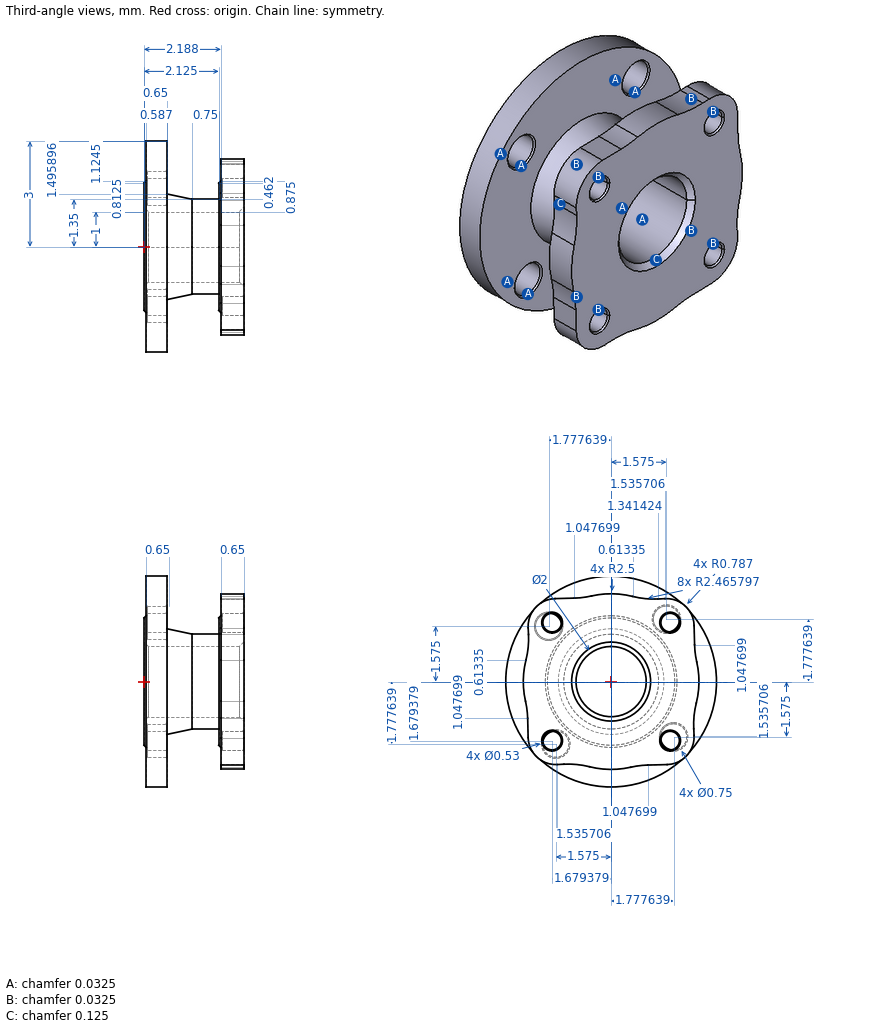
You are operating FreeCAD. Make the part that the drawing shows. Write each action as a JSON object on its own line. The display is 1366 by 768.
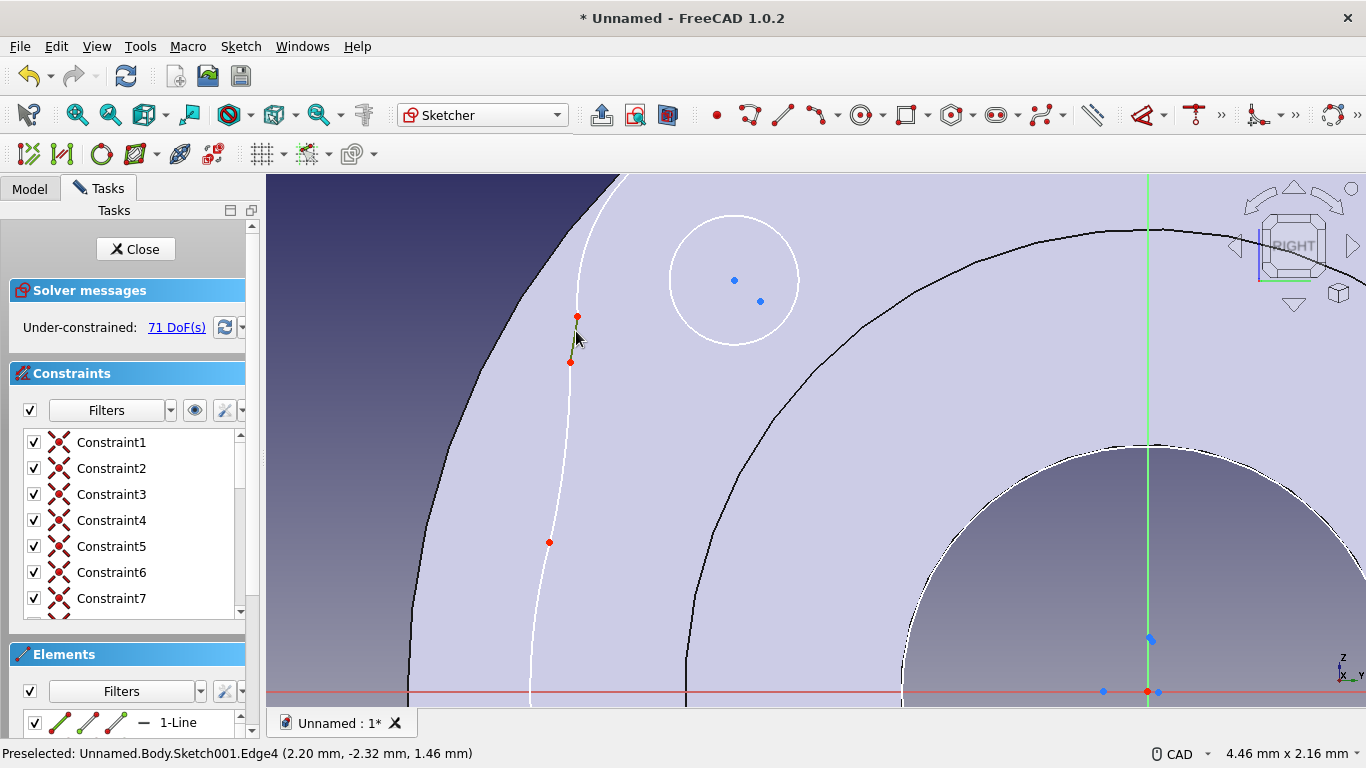
{"action": "scroll", "coordinate": [575, 332], "scroll_direction": "down", "scroll_amount": 6}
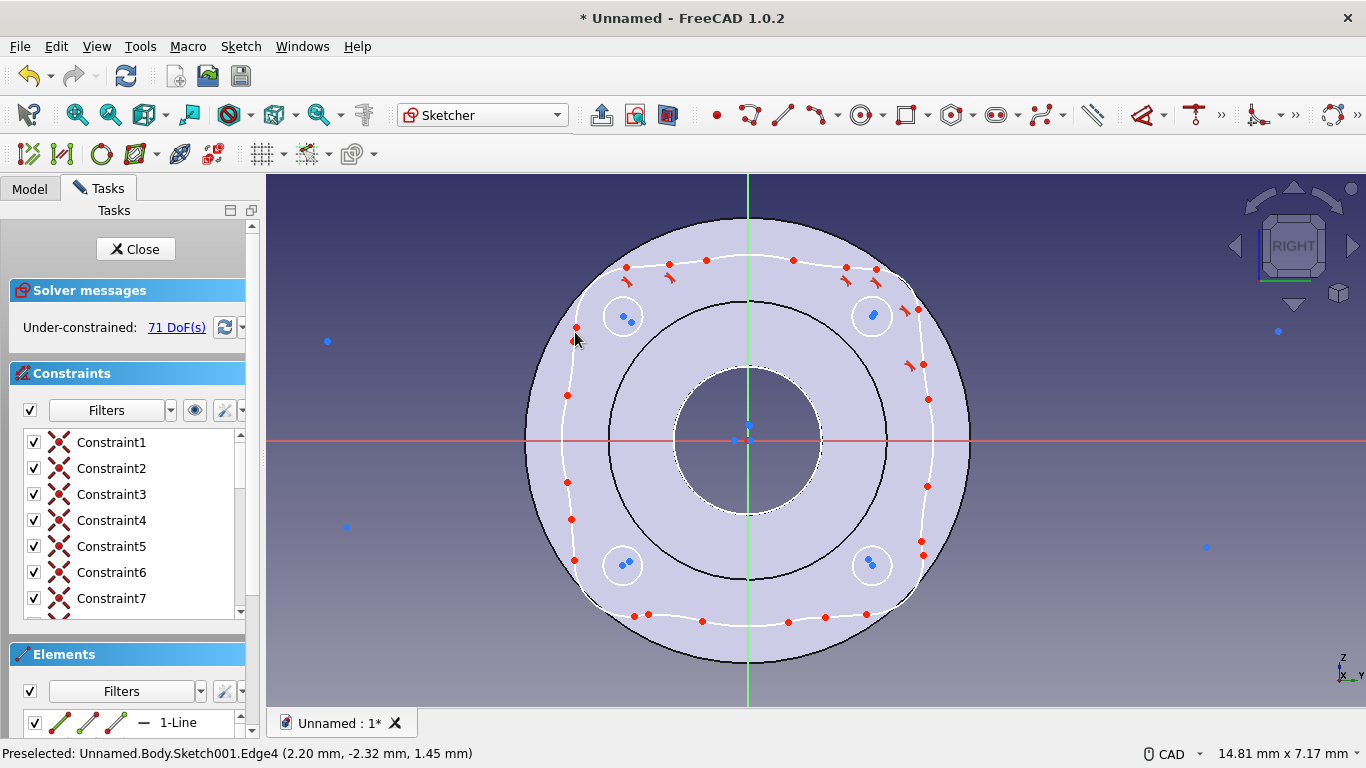
{"action": "left_click", "coordinate": [580, 302]}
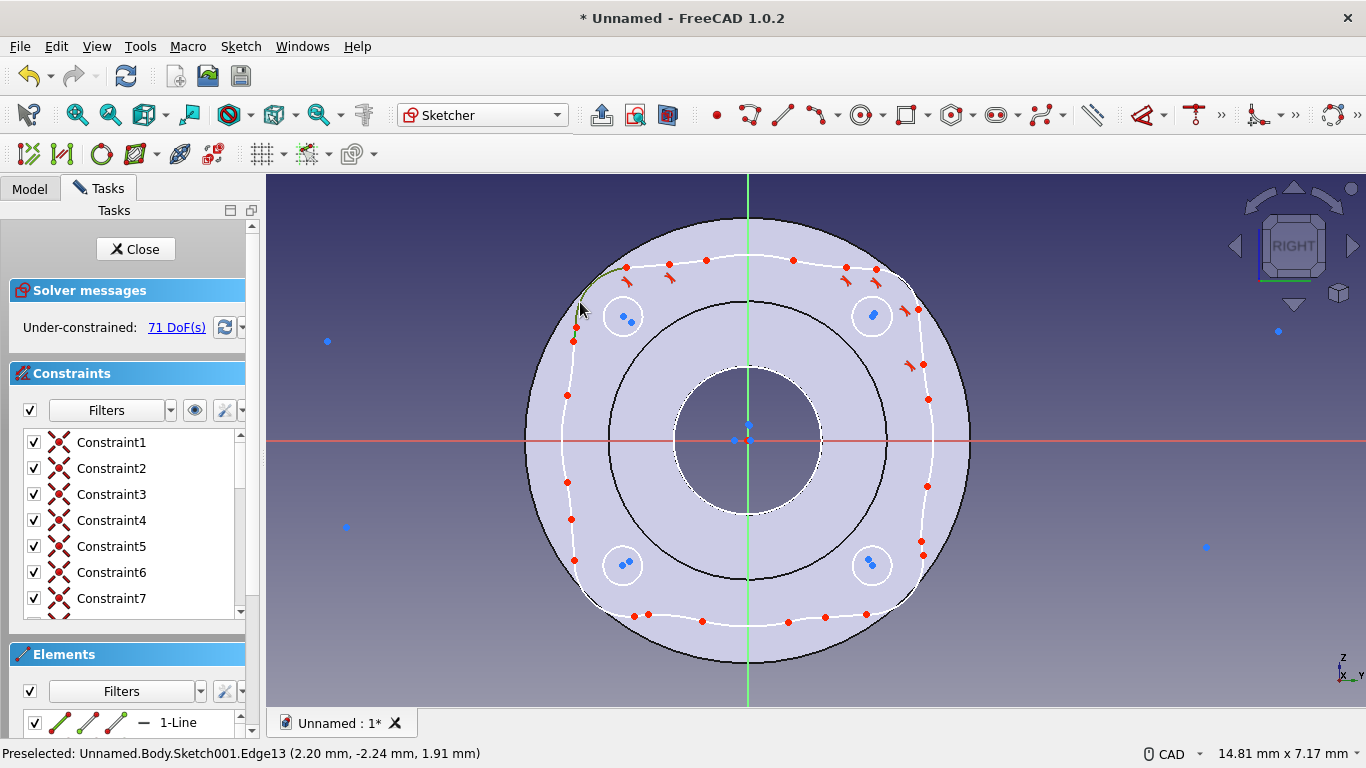
{"action": "key", "text": "t"}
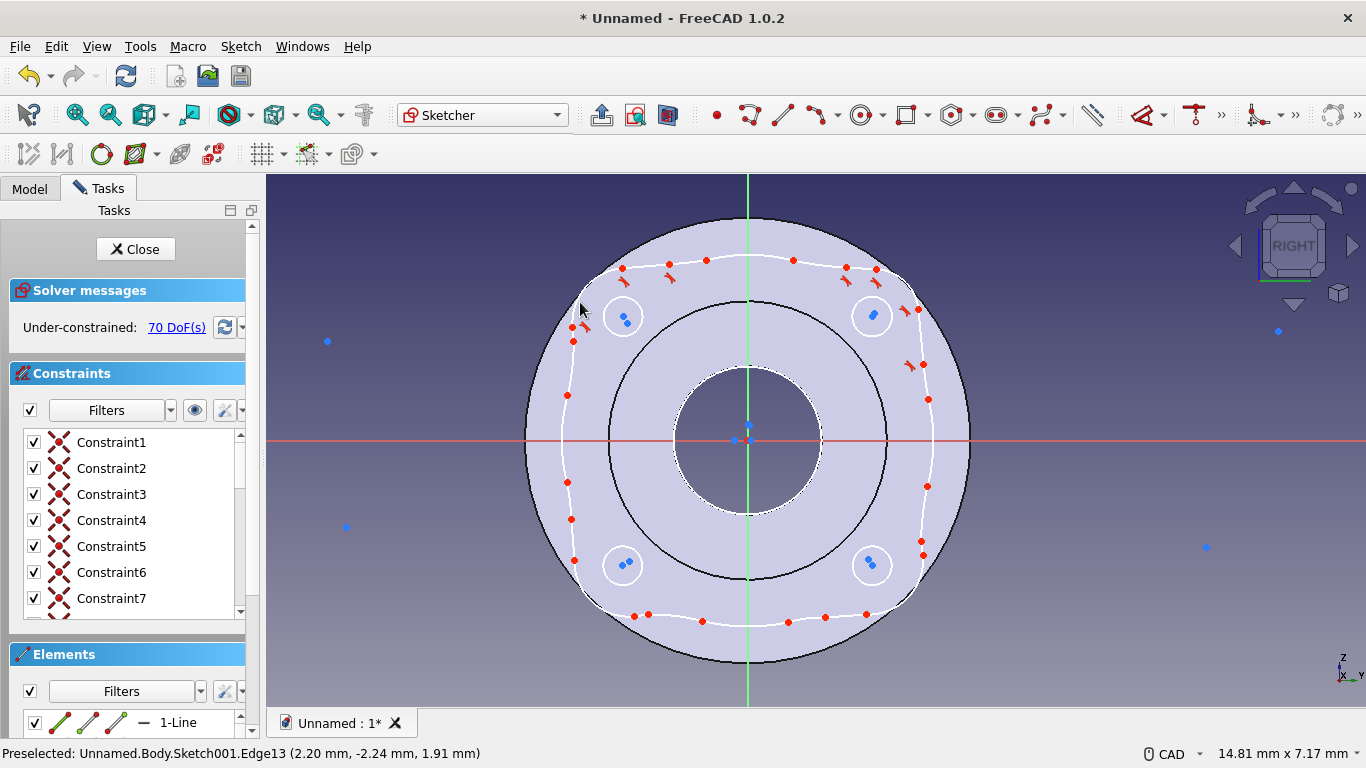
{"action": "scroll", "coordinate": [573, 335], "scroll_direction": "up", "scroll_amount": 4}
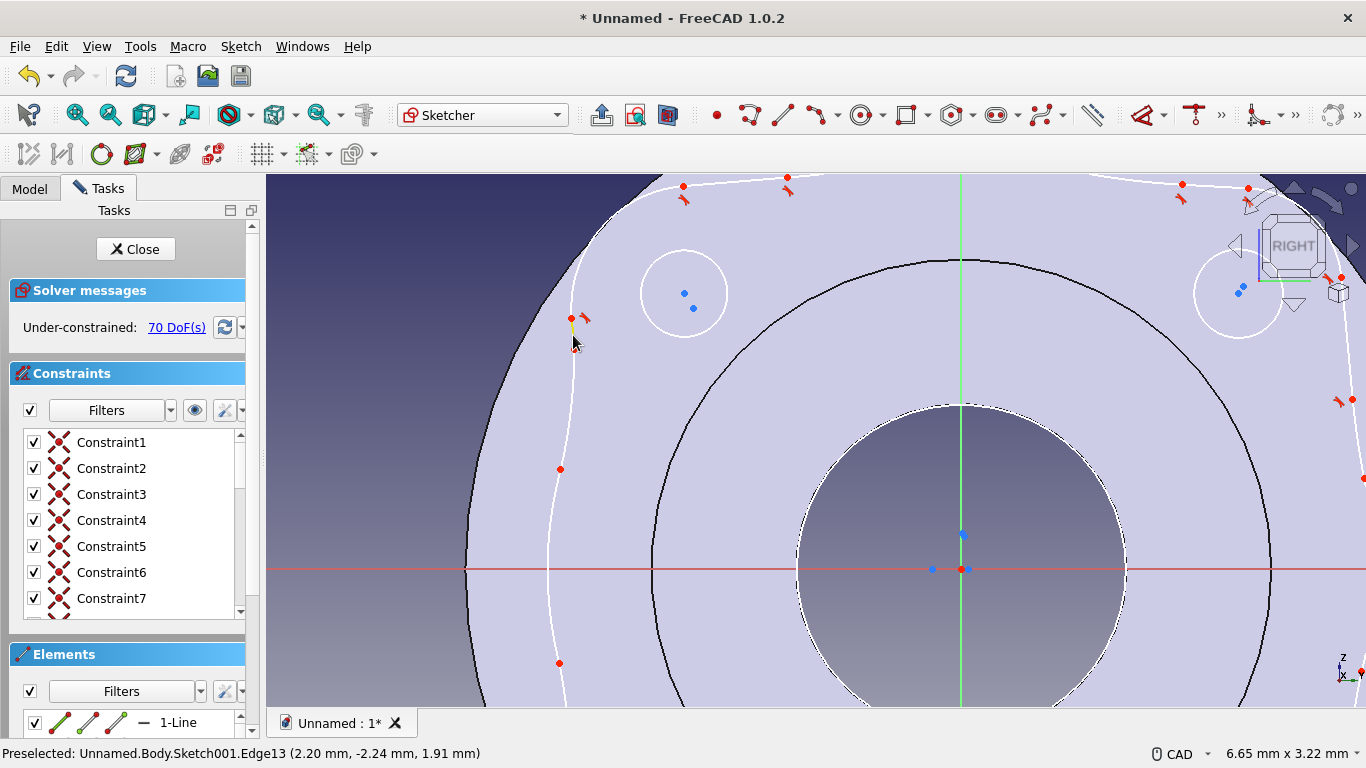
{"action": "left_click", "coordinate": [573, 334]}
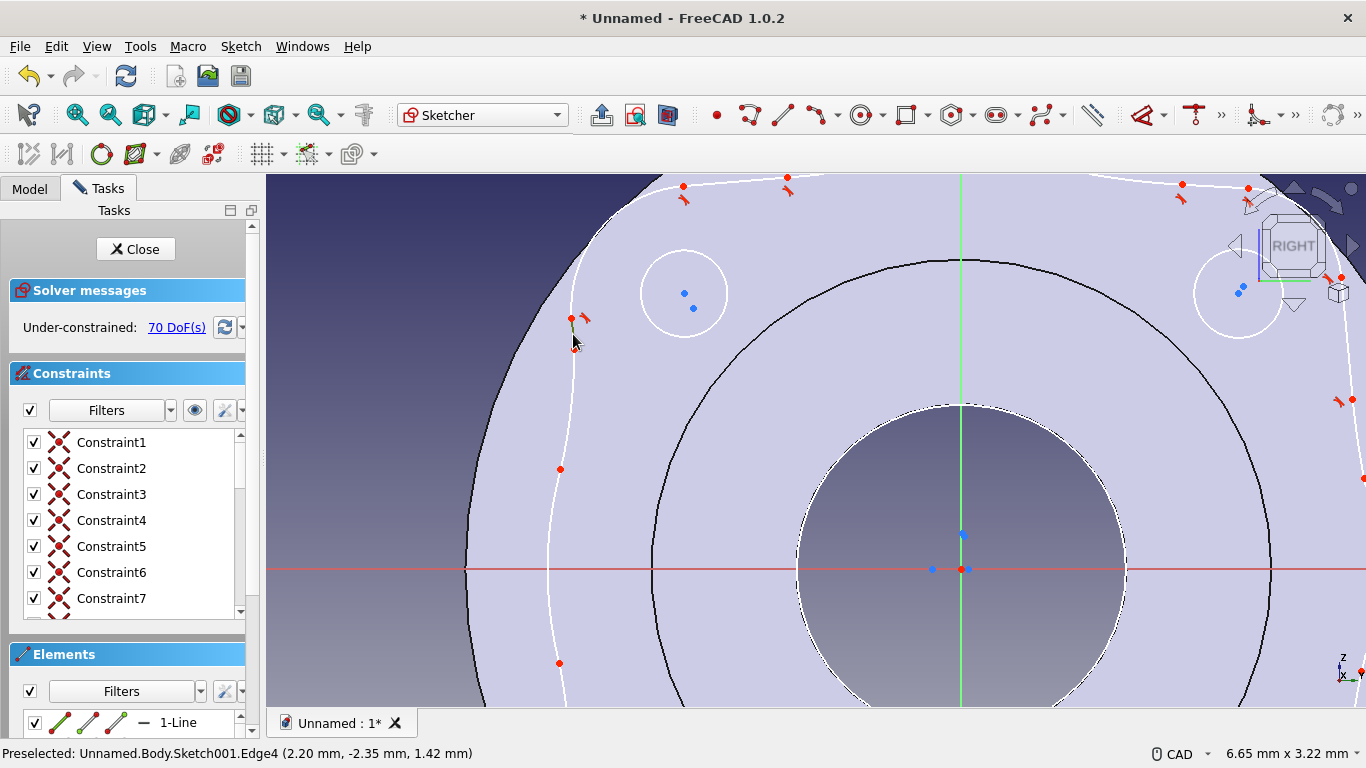
{"action": "left_click", "coordinate": [568, 434]}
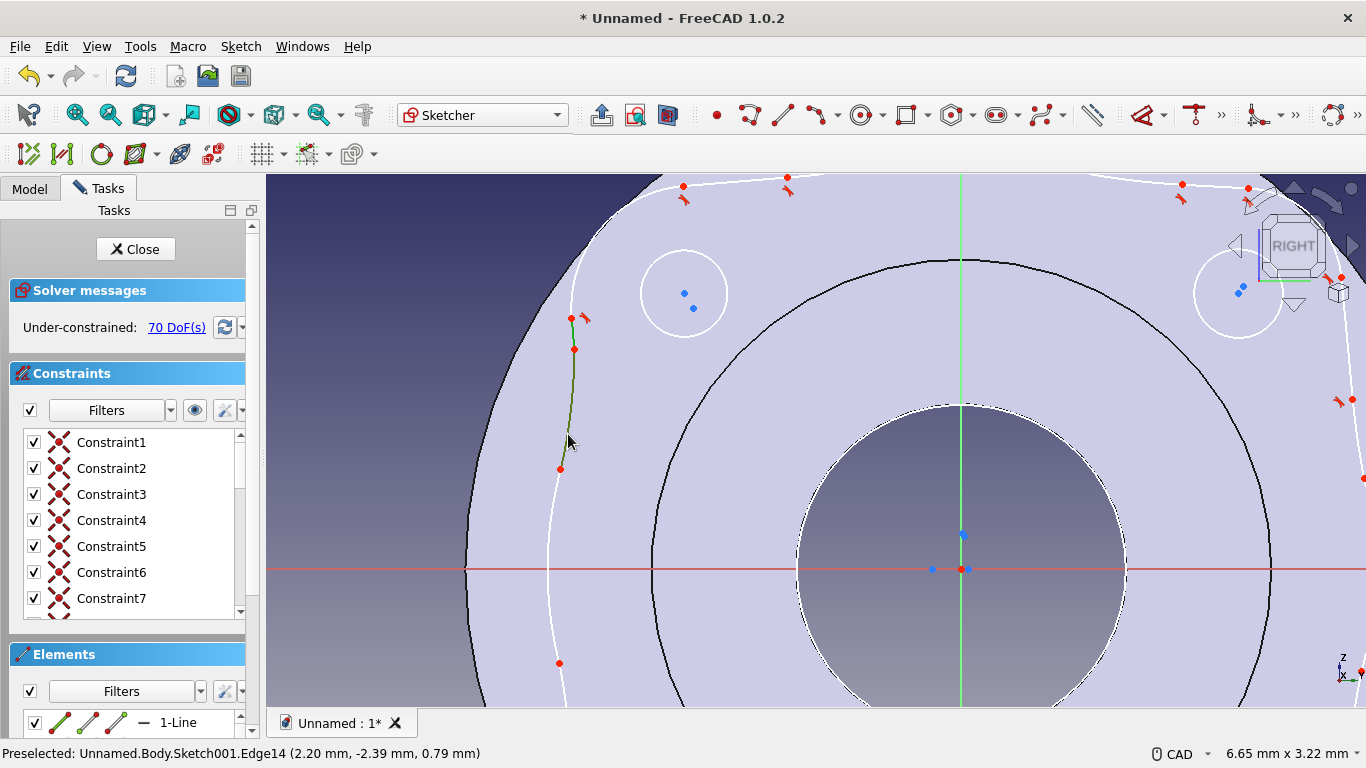
{"action": "key", "text": "t"}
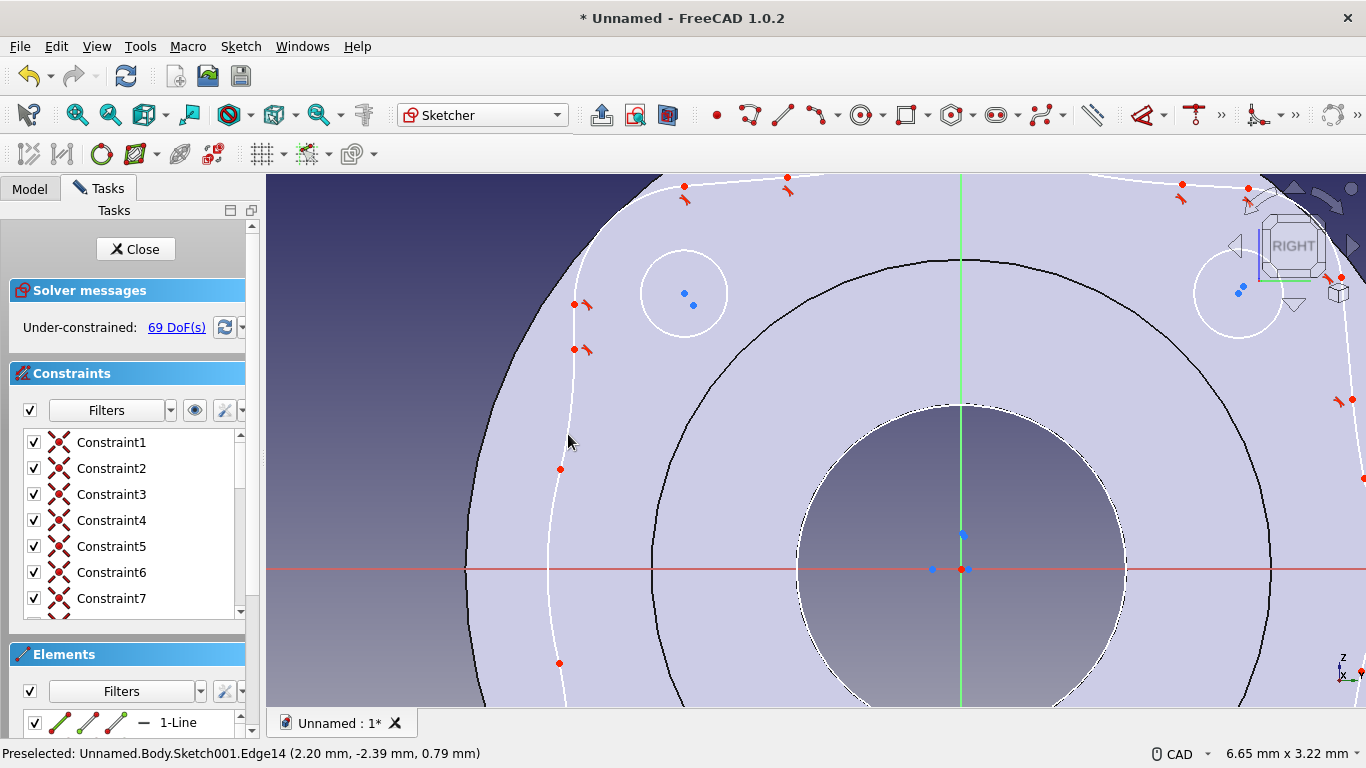
{"action": "scroll", "coordinate": [573, 335], "scroll_direction": "down", "scroll_amount": 4}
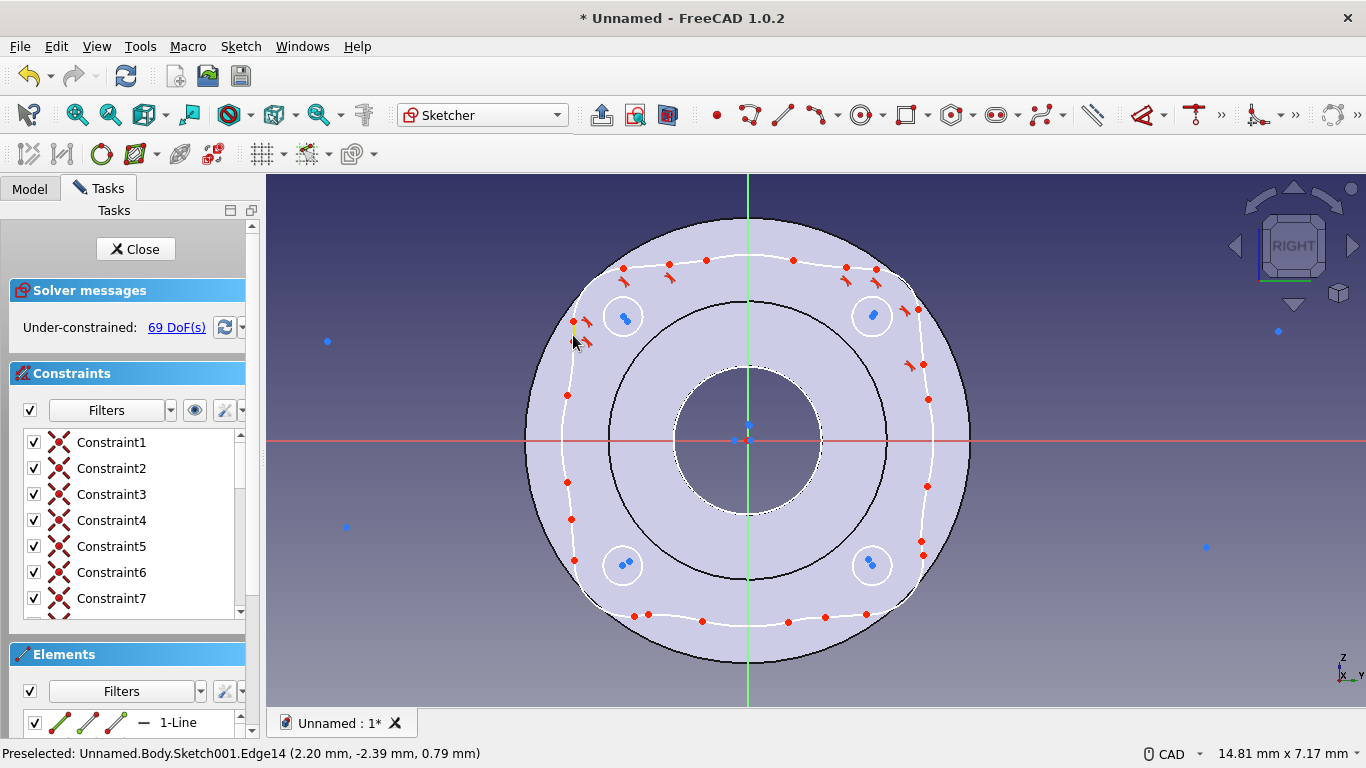
{"action": "left_click", "coordinate": [572, 531]}